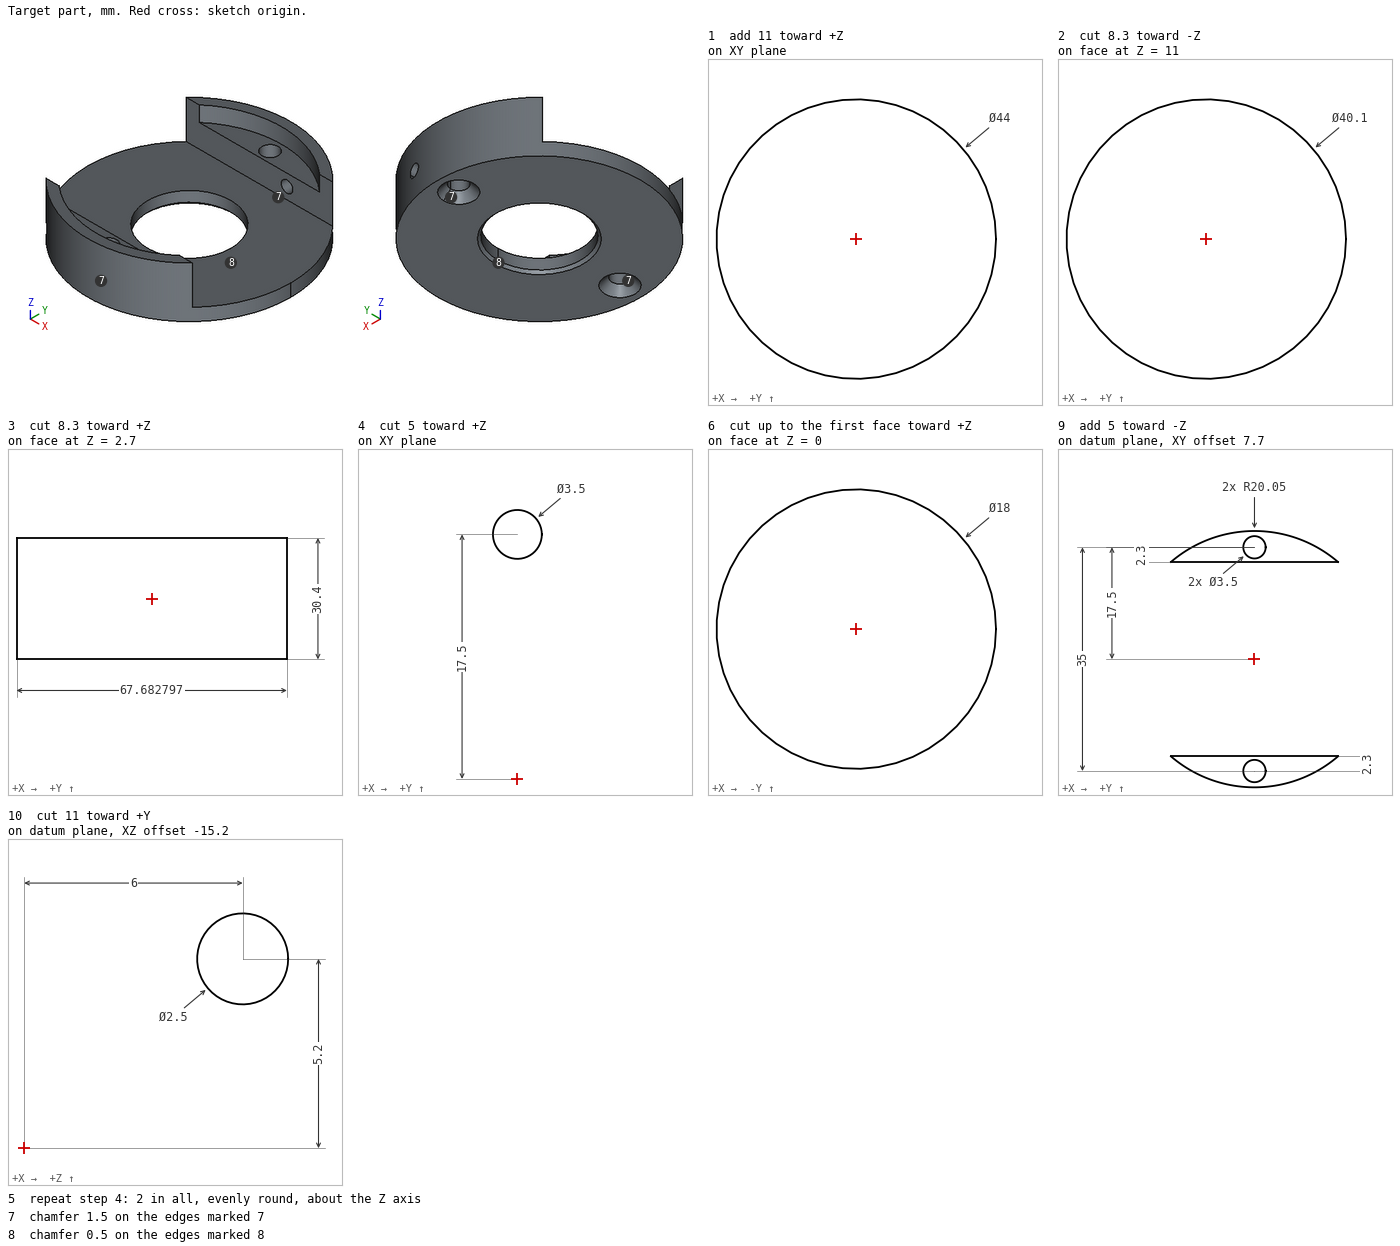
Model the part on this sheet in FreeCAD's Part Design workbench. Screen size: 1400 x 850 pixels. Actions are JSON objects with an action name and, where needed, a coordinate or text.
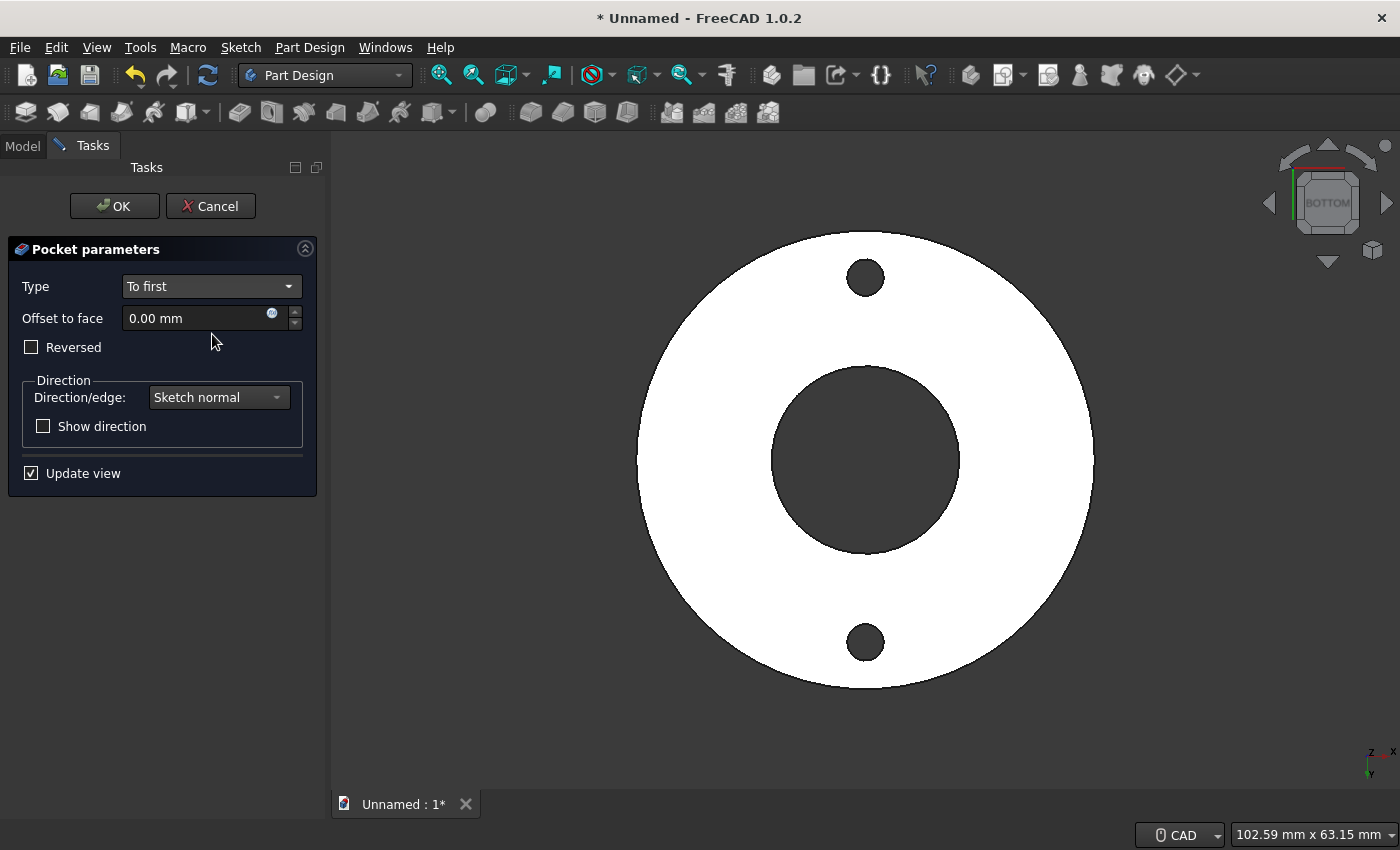
{"action": "left_click", "coordinate": [115, 206]}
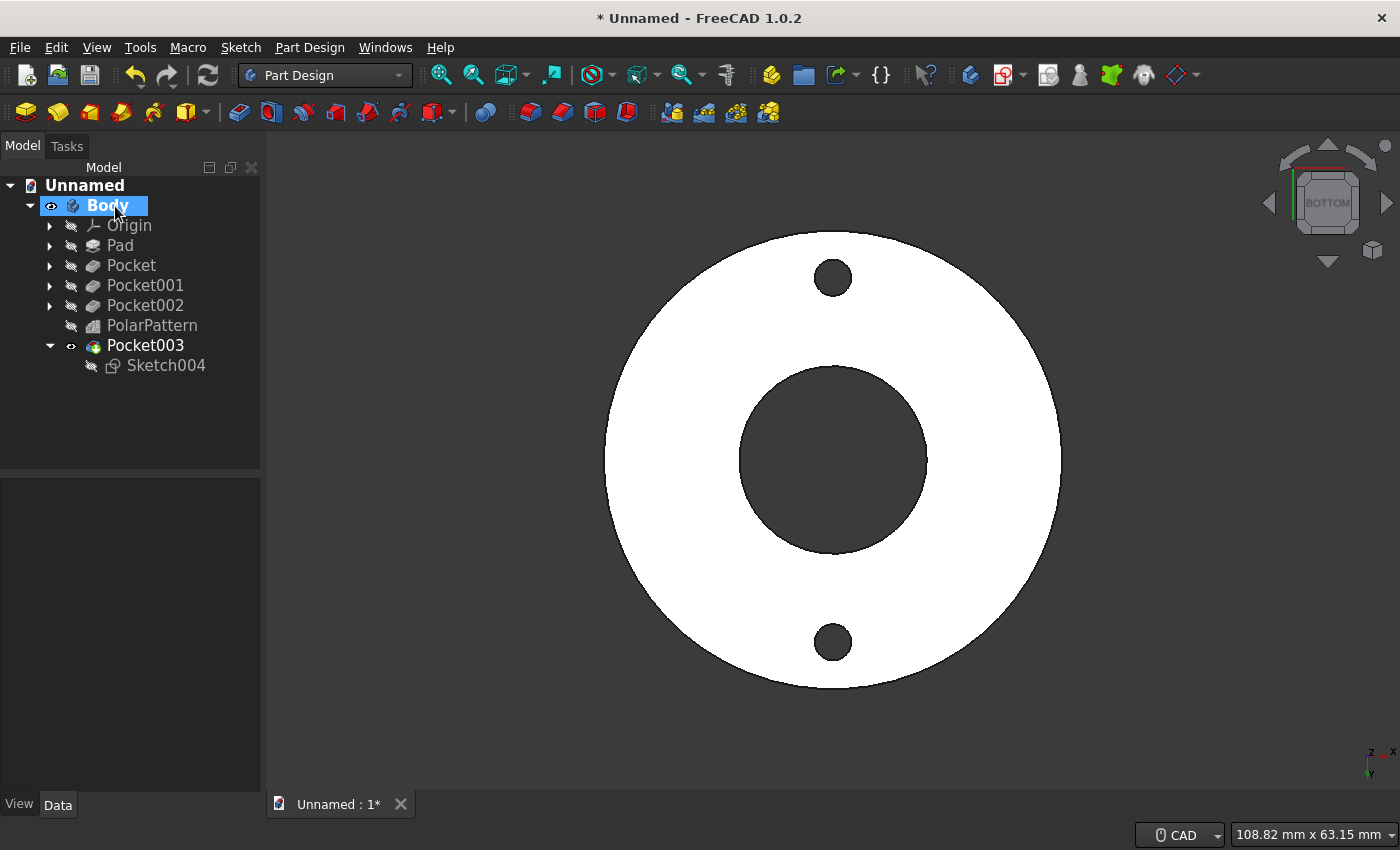
{"action": "left_click", "coordinate": [815, 641]}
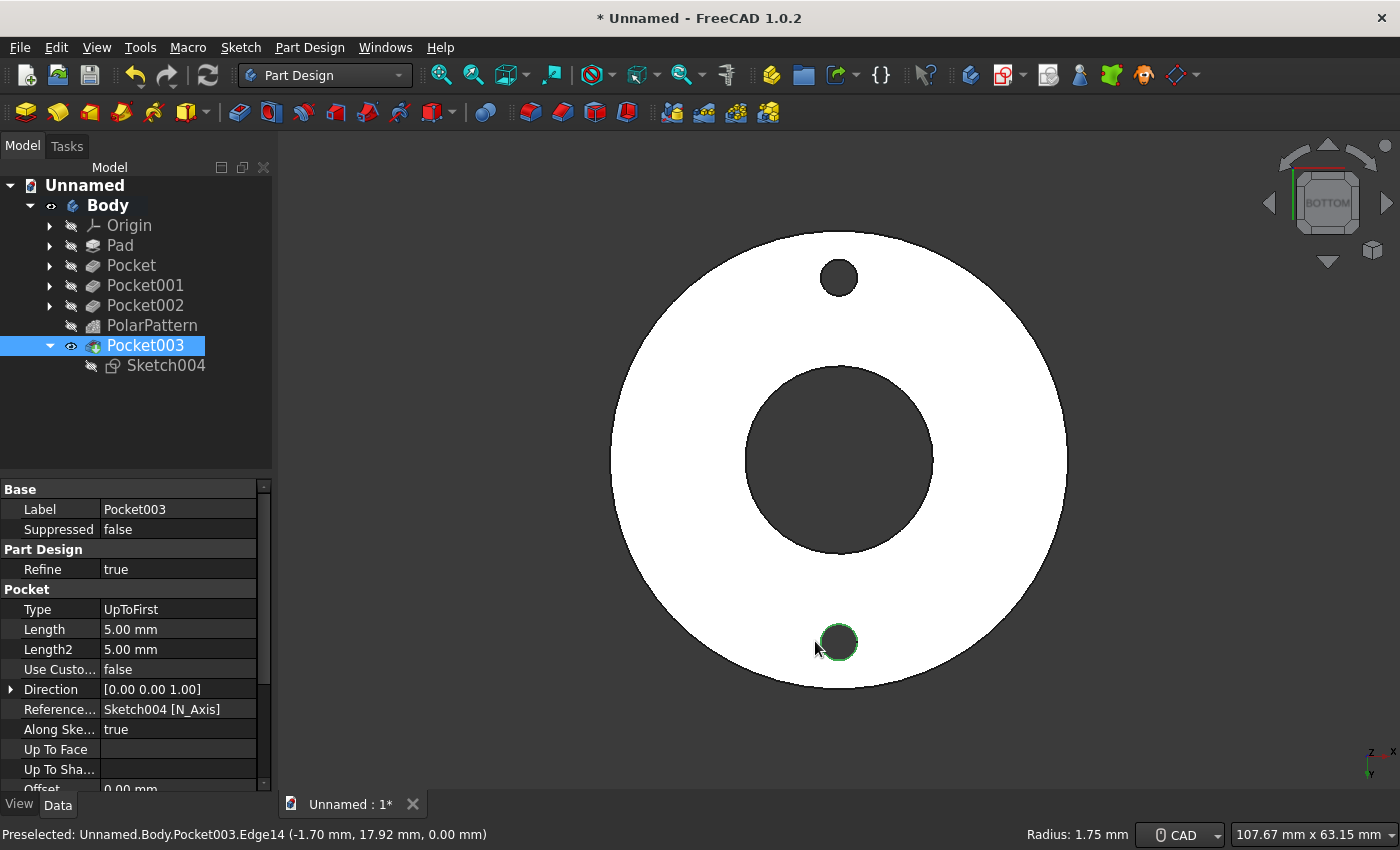
{"action": "left_click", "coordinate": [857, 277], "text": "ctrl"}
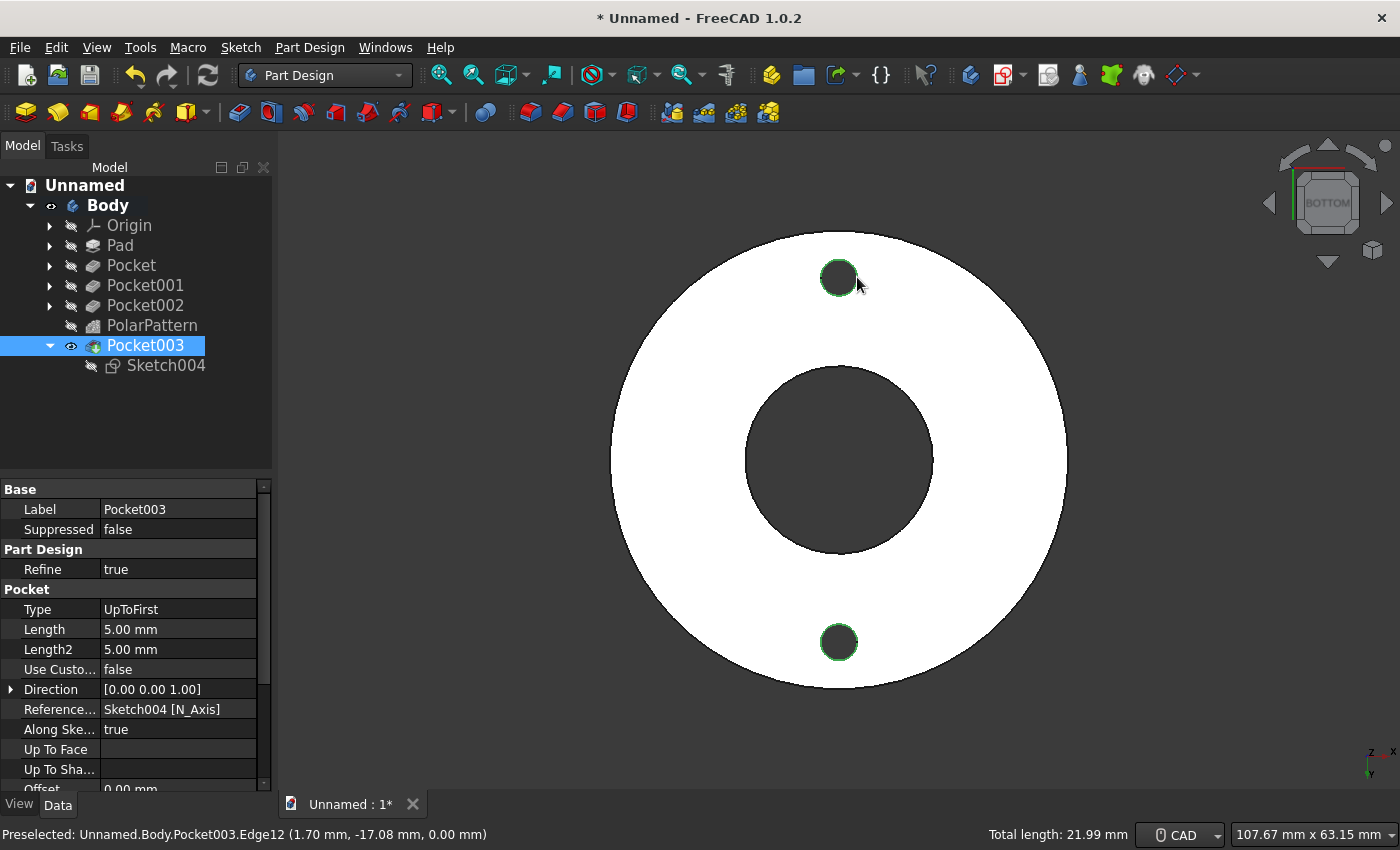
{"action": "left_click", "coordinate": [564, 112]}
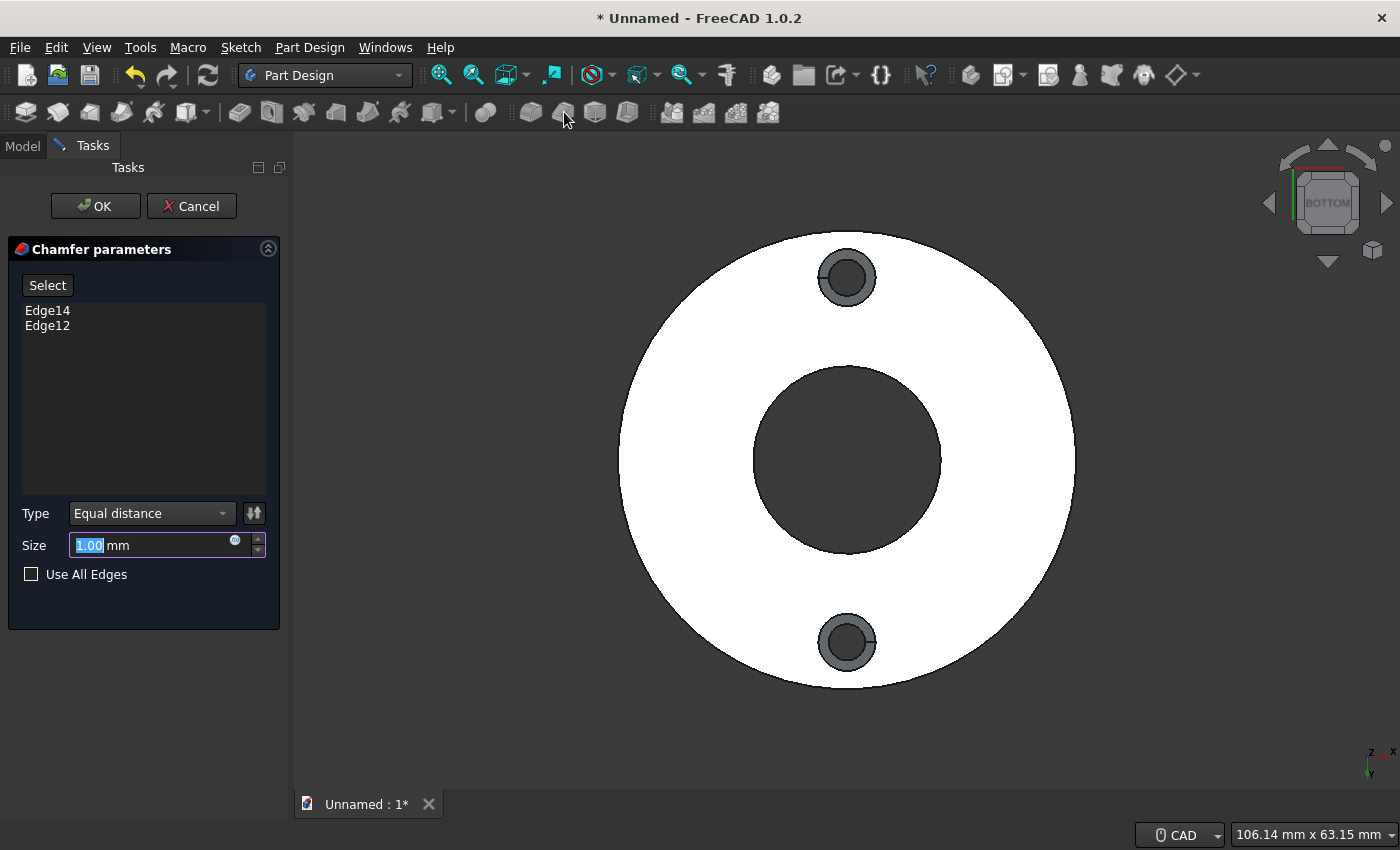
{"action": "type", "text": "1.5"}
{"action": "key", "text": "Tab"}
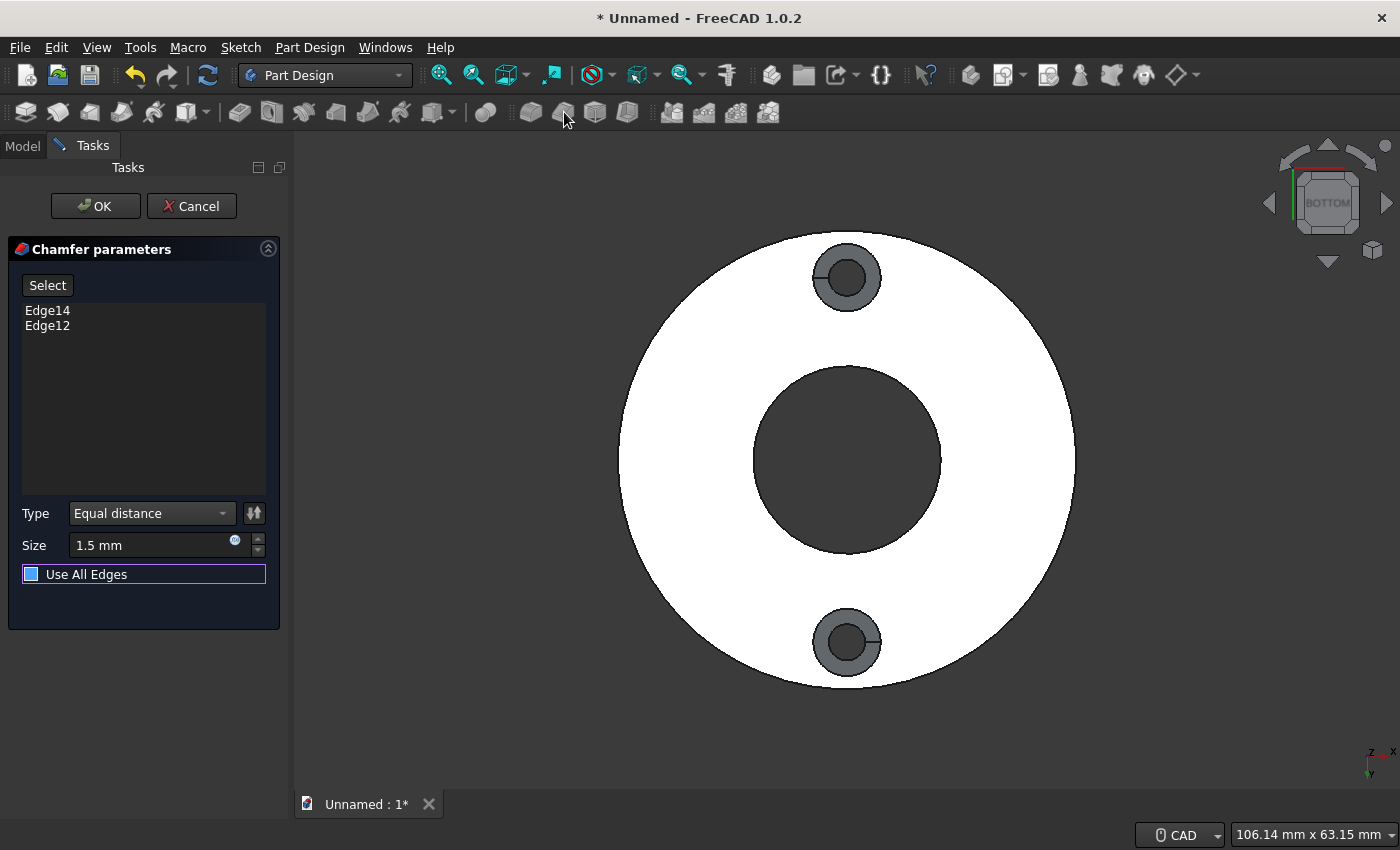
{"action": "left_click", "coordinate": [96, 206]}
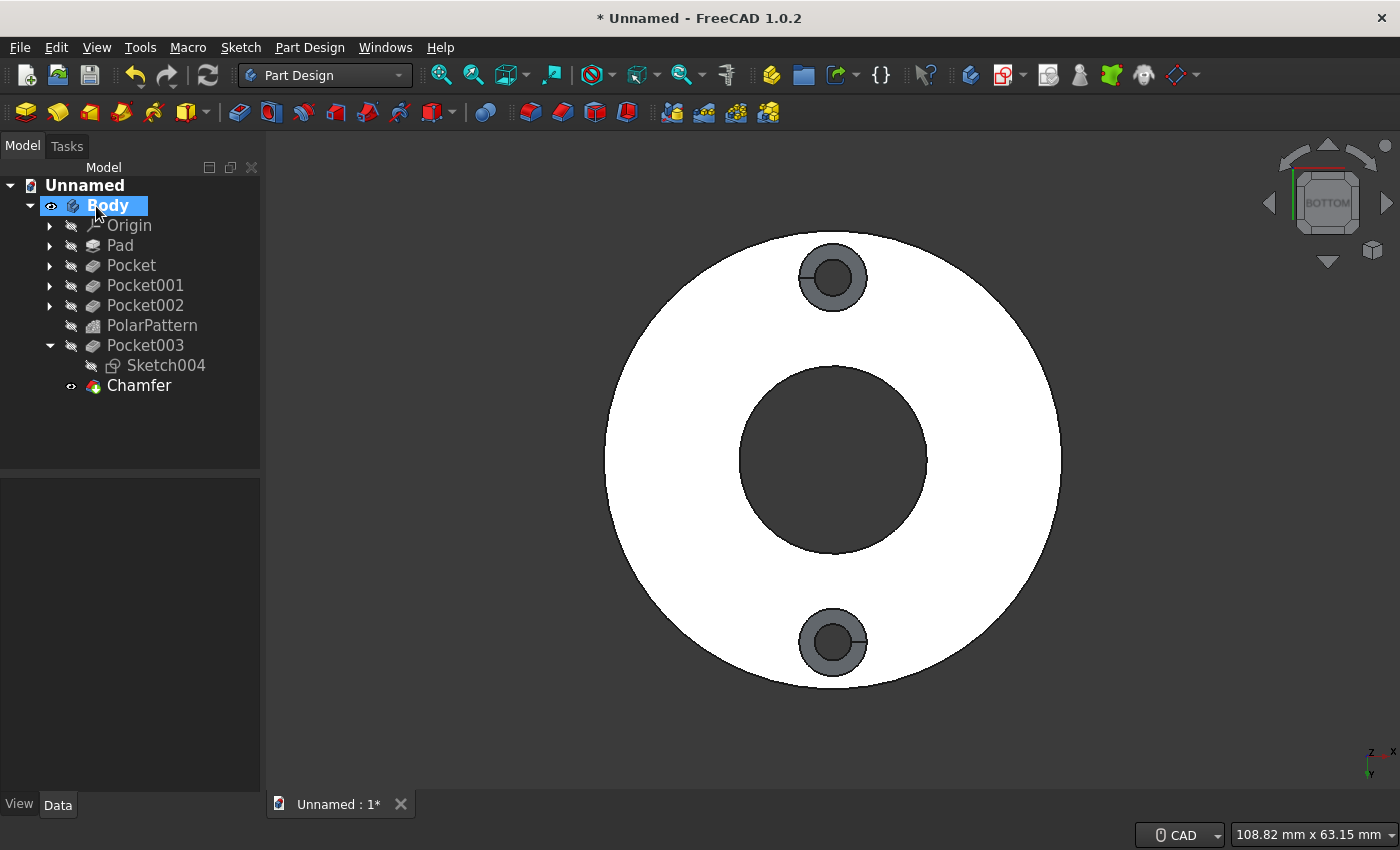
{"action": "left_click", "coordinate": [757, 404]}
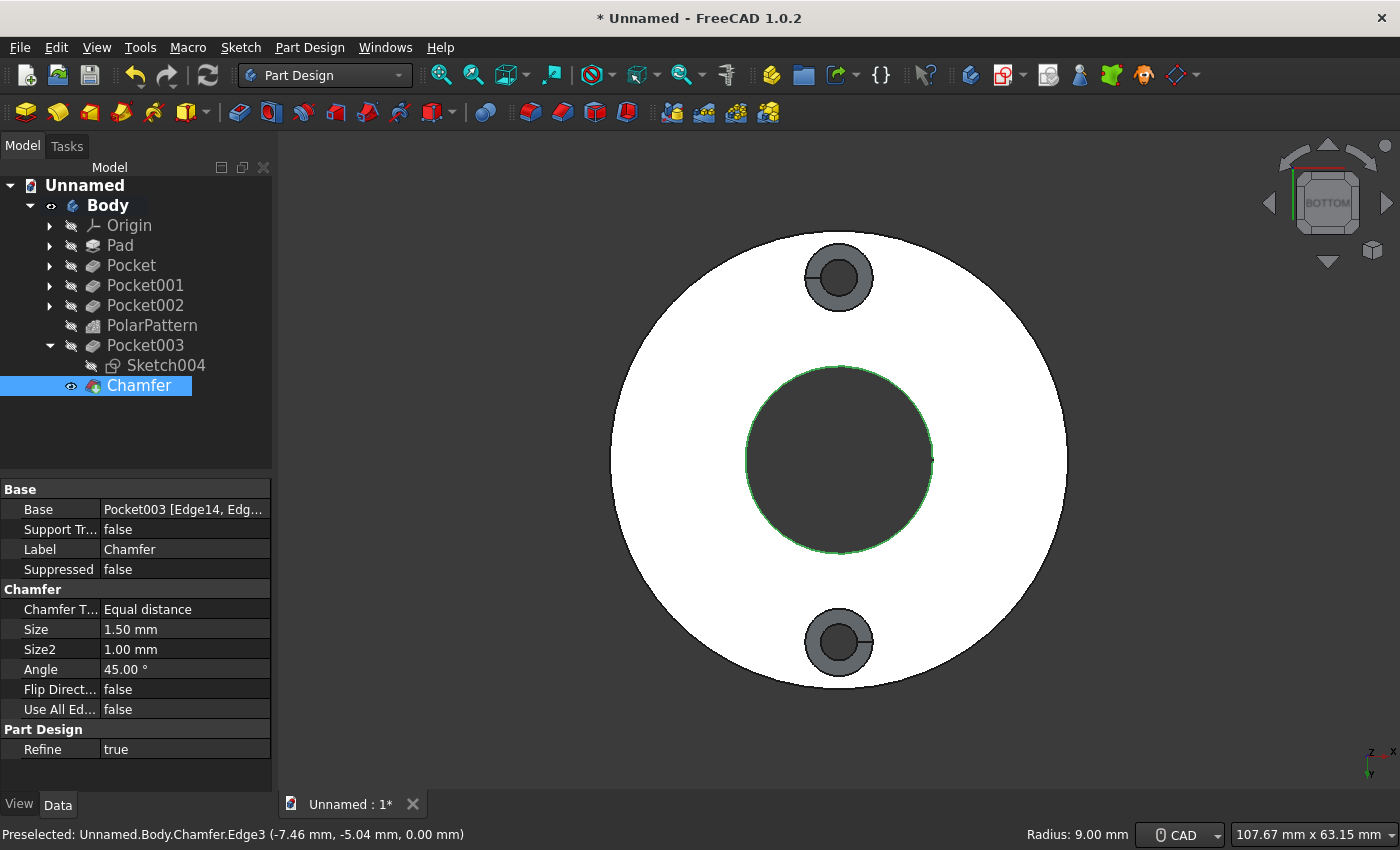
{"action": "left_click", "coordinate": [564, 112]}